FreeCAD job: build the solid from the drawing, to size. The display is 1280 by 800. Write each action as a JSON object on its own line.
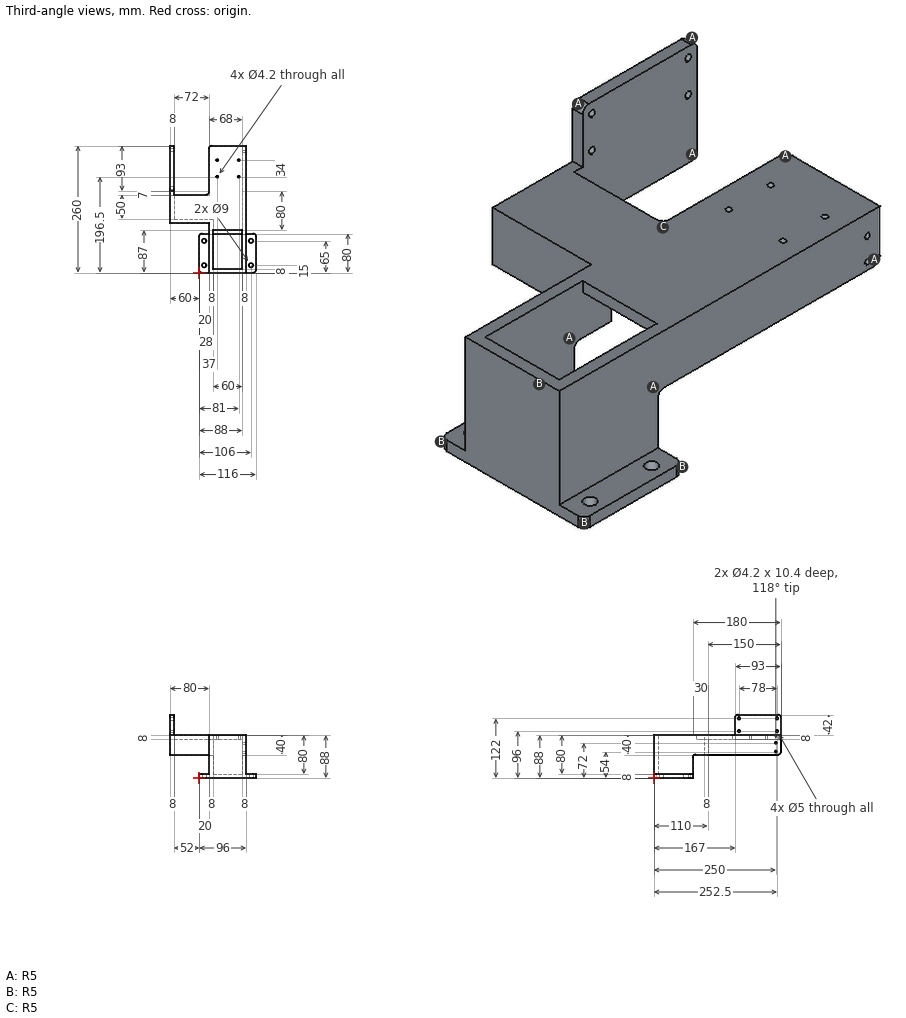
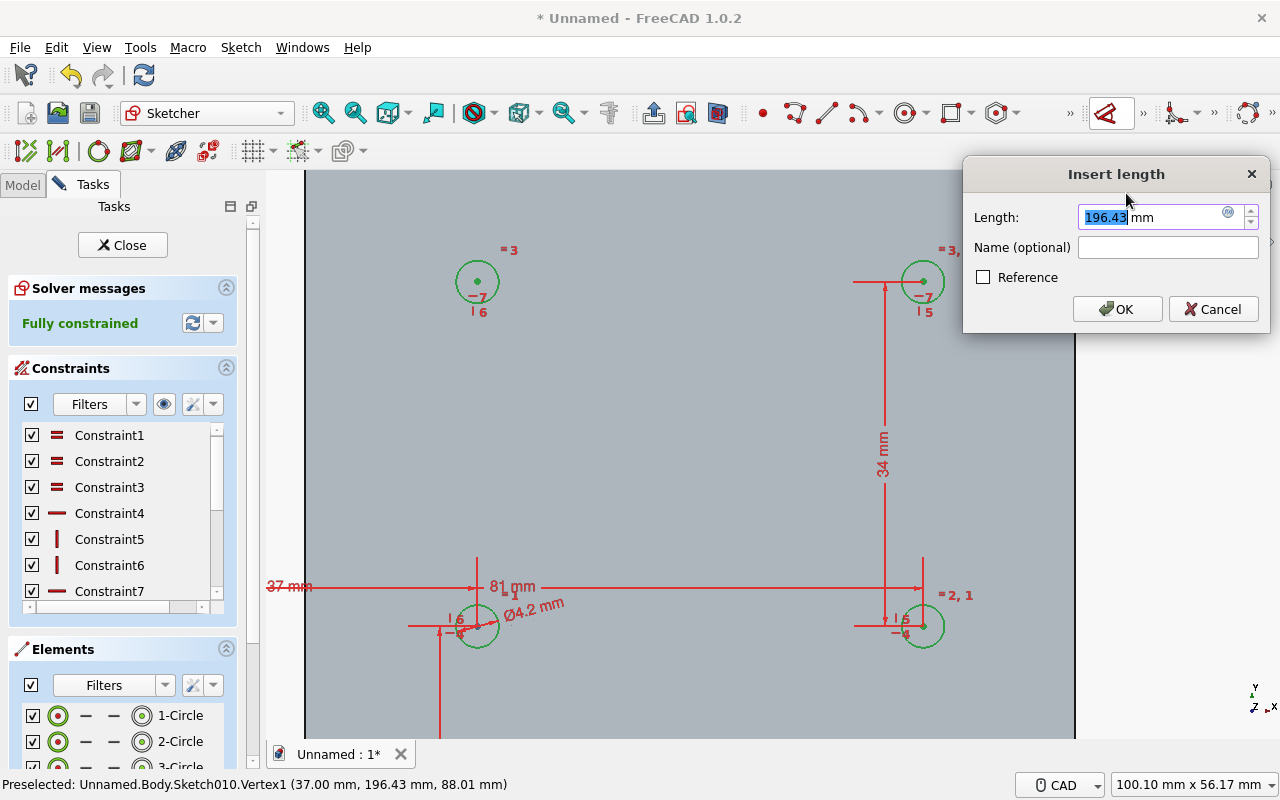
{"action": "type", "text": "196.5"}
{"action": "key", "text": "Return"}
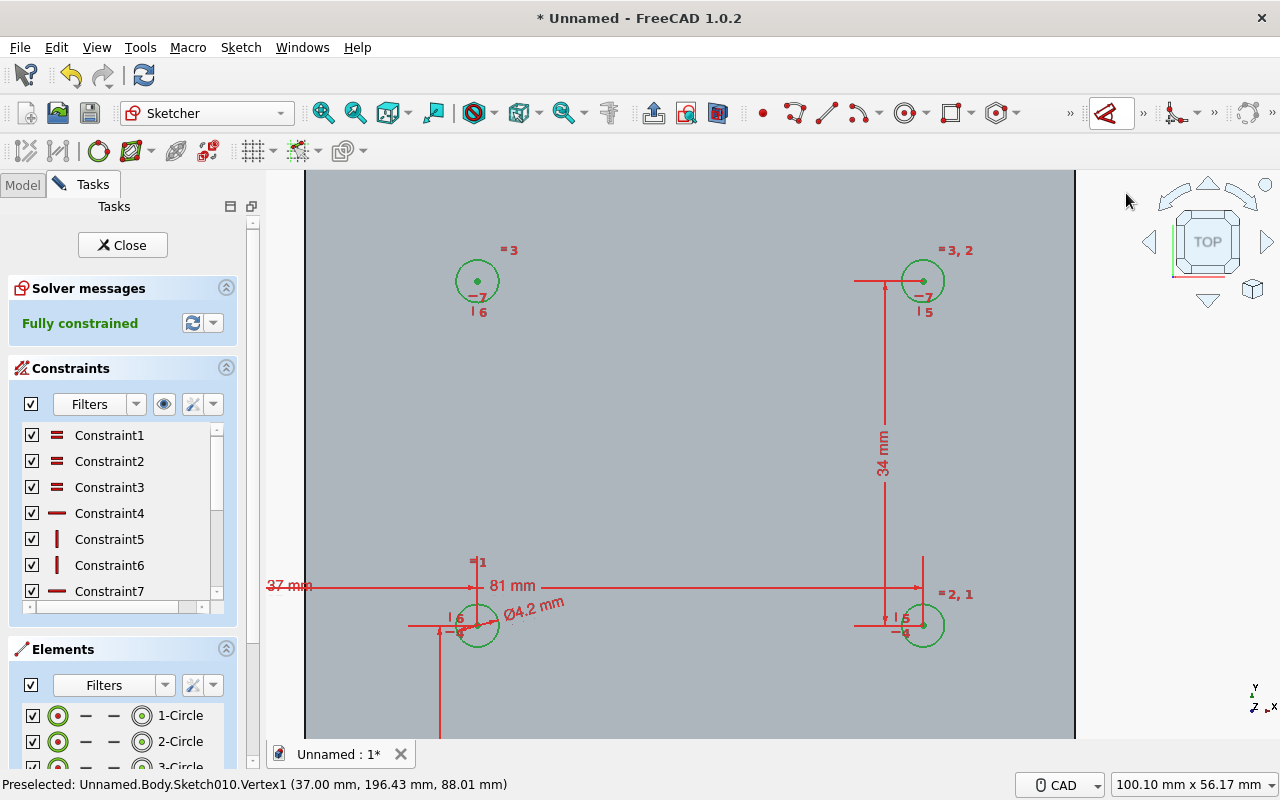
{"action": "left_click", "coordinate": [123, 245]}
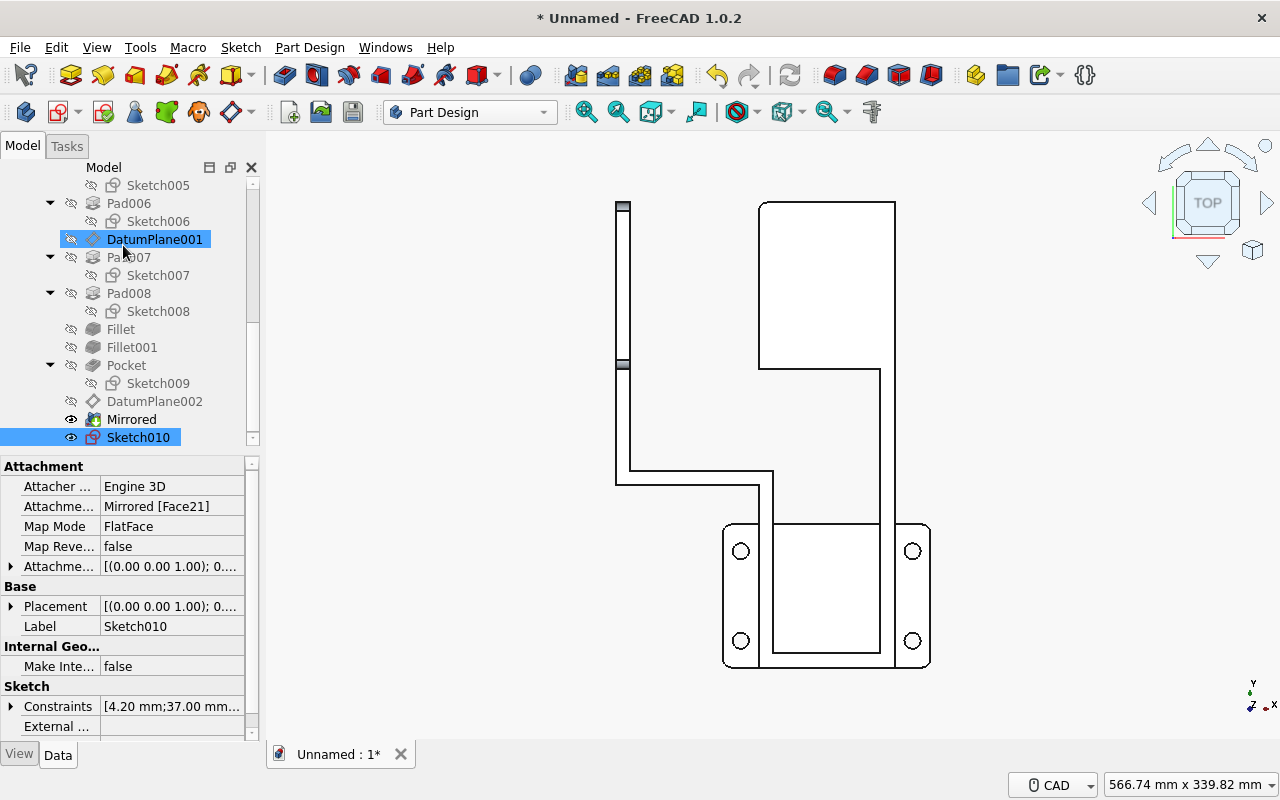
{"action": "left_click", "coordinate": [318, 76]}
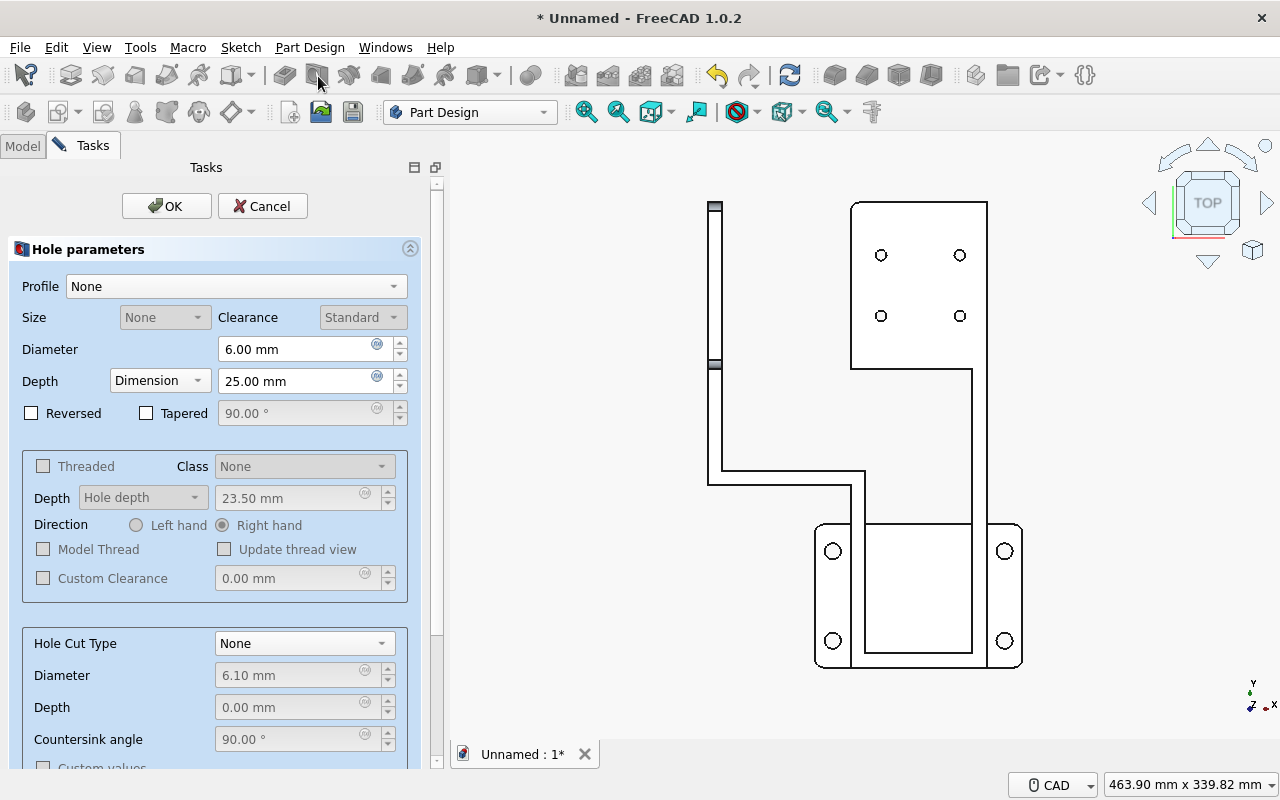
{"action": "triple_click", "coordinate": [305, 349]}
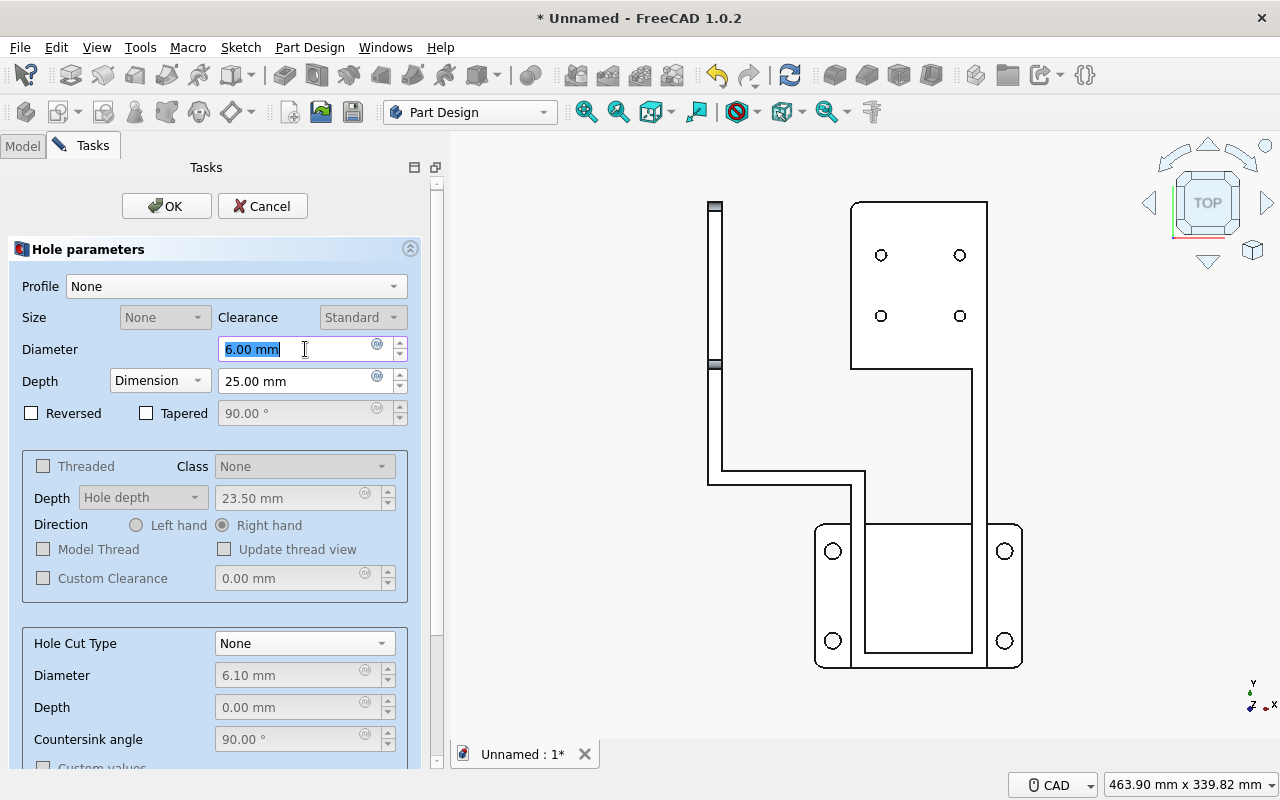
{"action": "type", "text": "4.2"}
{"action": "key", "text": "Tab"}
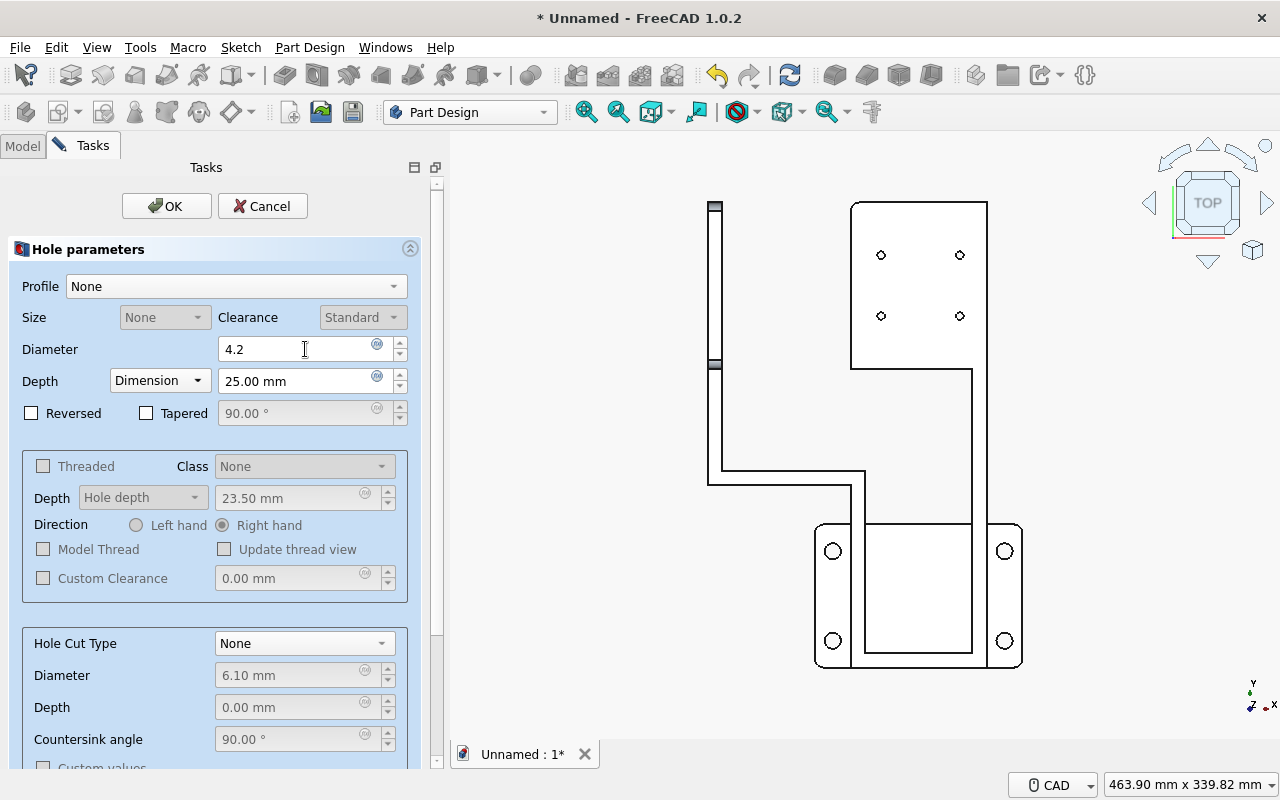
{"action": "left_click", "coordinate": [161, 380]}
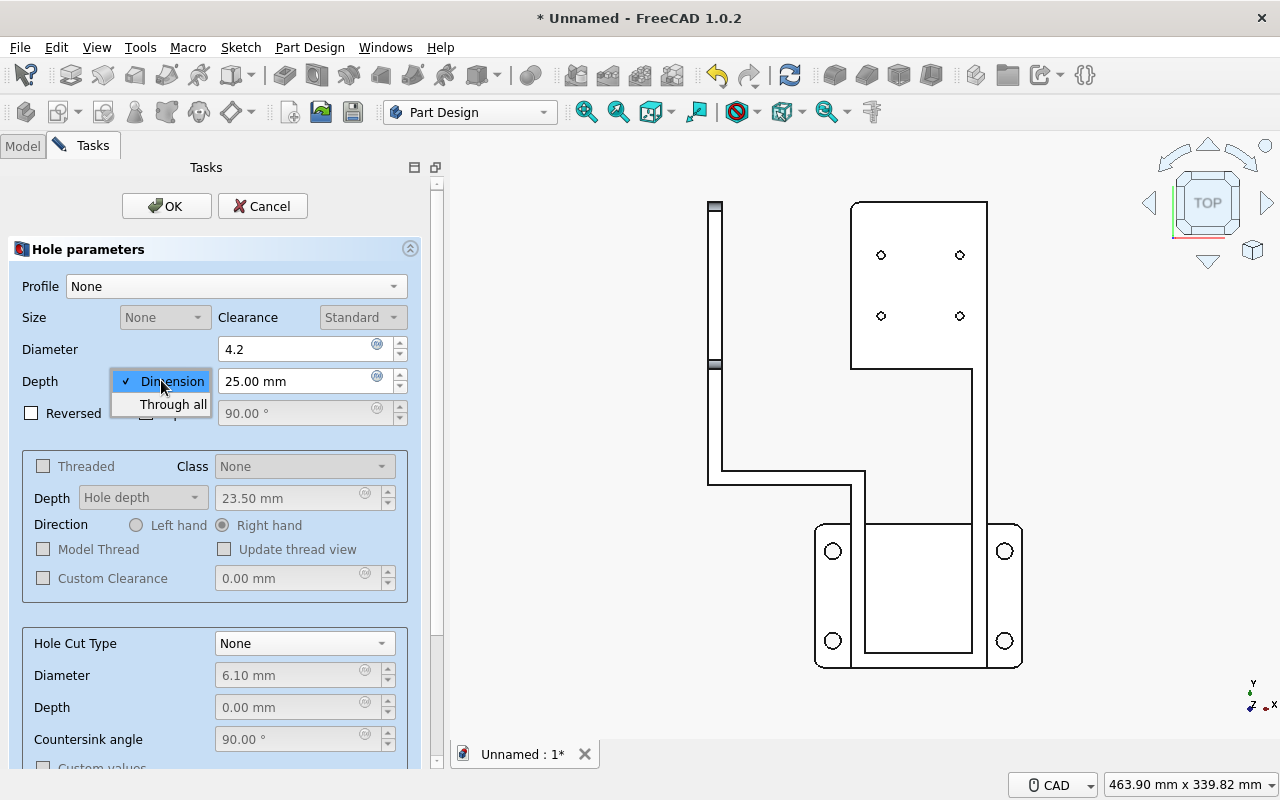
{"action": "left_click", "coordinate": [160, 404]}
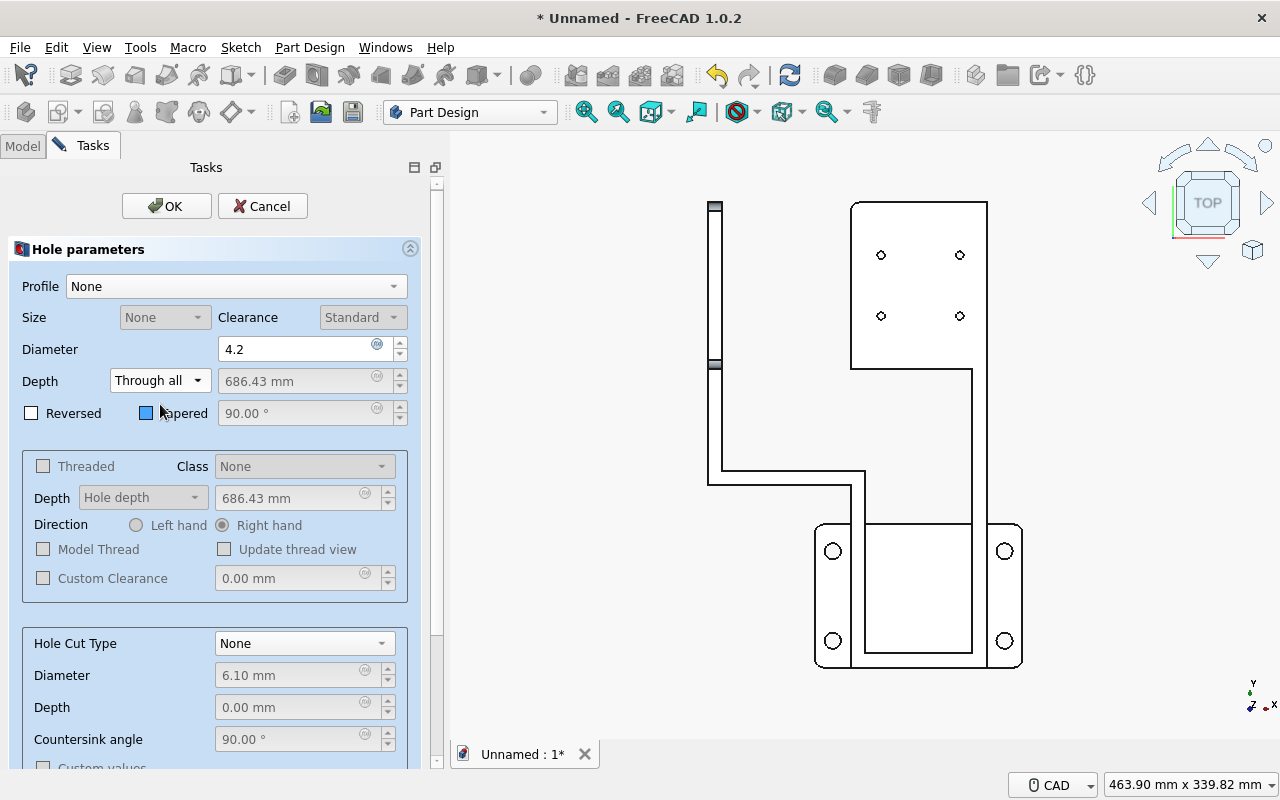
{"action": "left_click", "coordinate": [167, 206]}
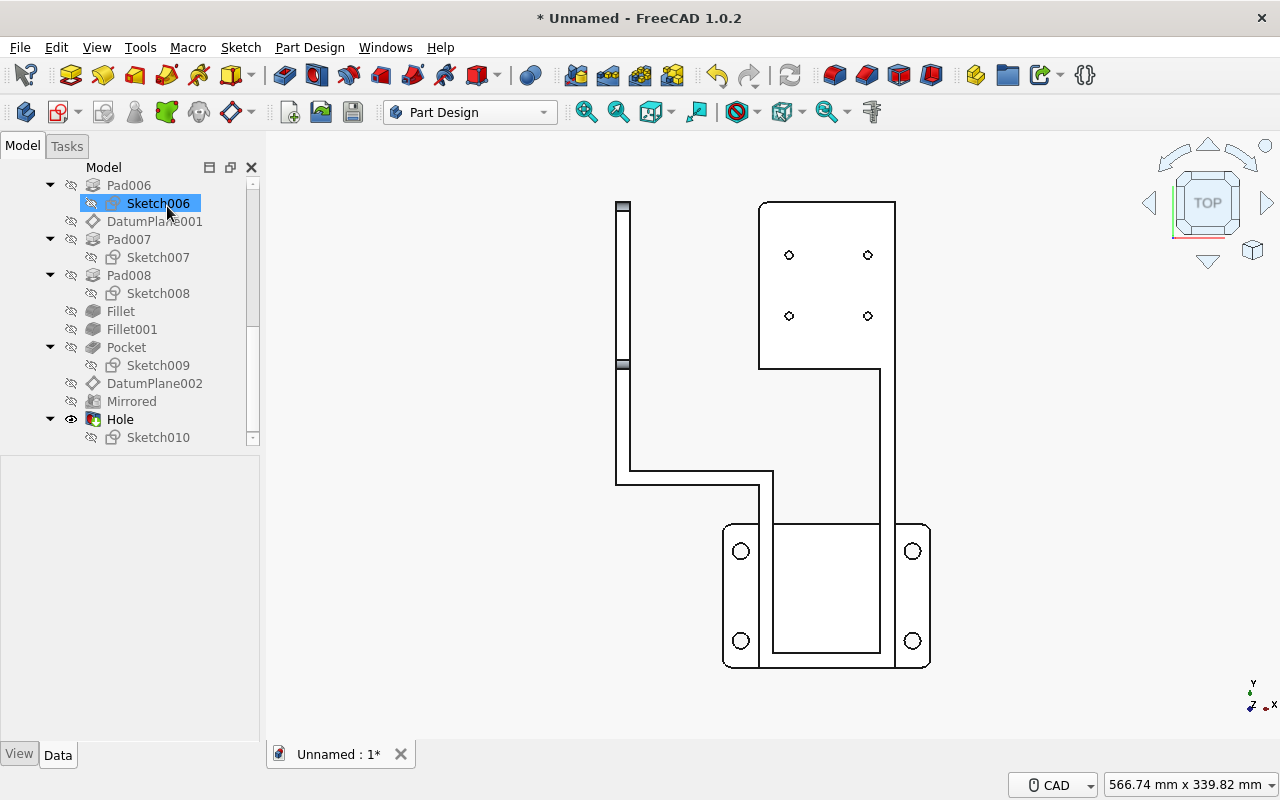
{"action": "key", "text": "0"}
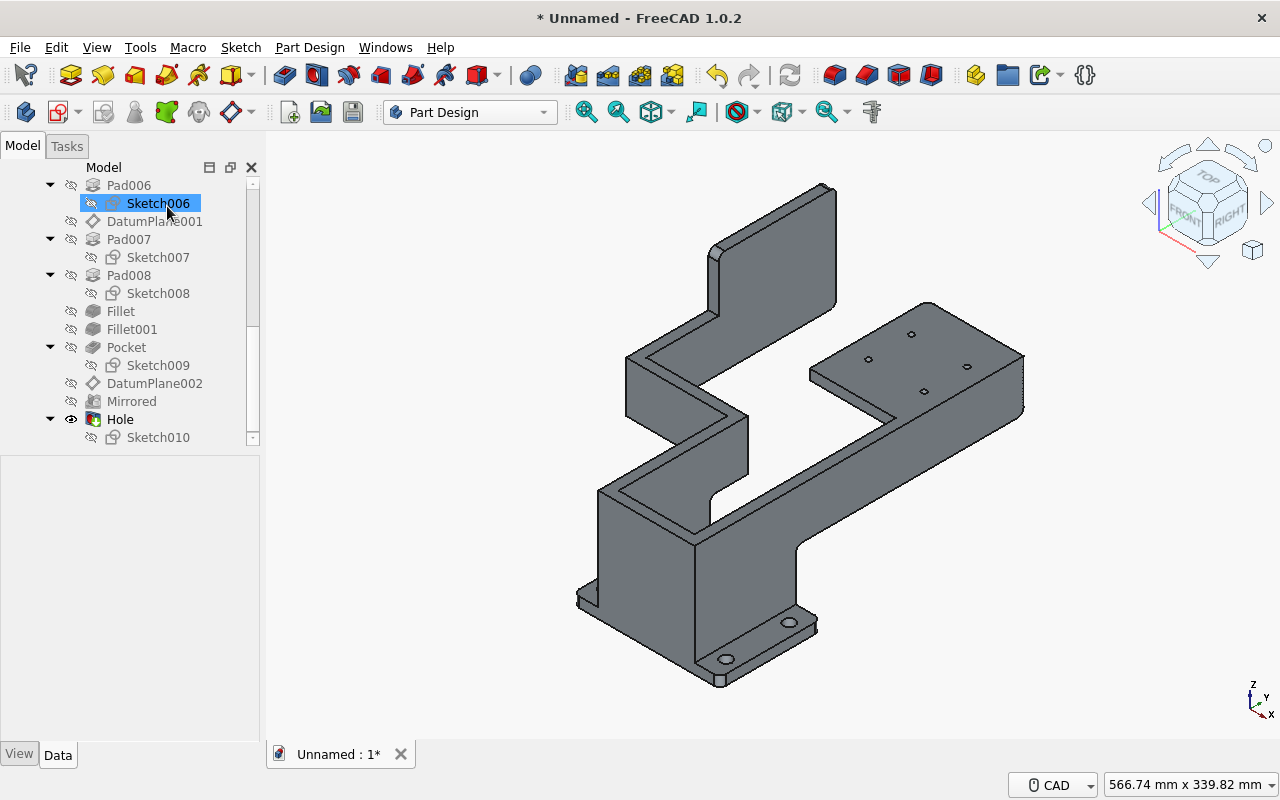
{"action": "left_click", "coordinate": [768, 285]}